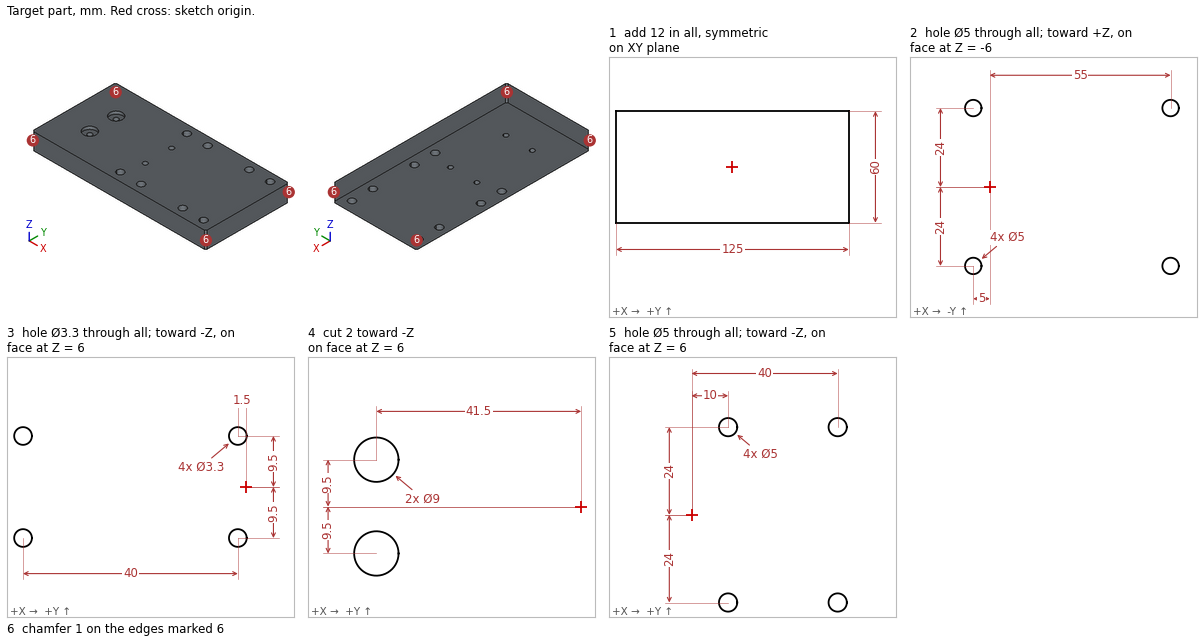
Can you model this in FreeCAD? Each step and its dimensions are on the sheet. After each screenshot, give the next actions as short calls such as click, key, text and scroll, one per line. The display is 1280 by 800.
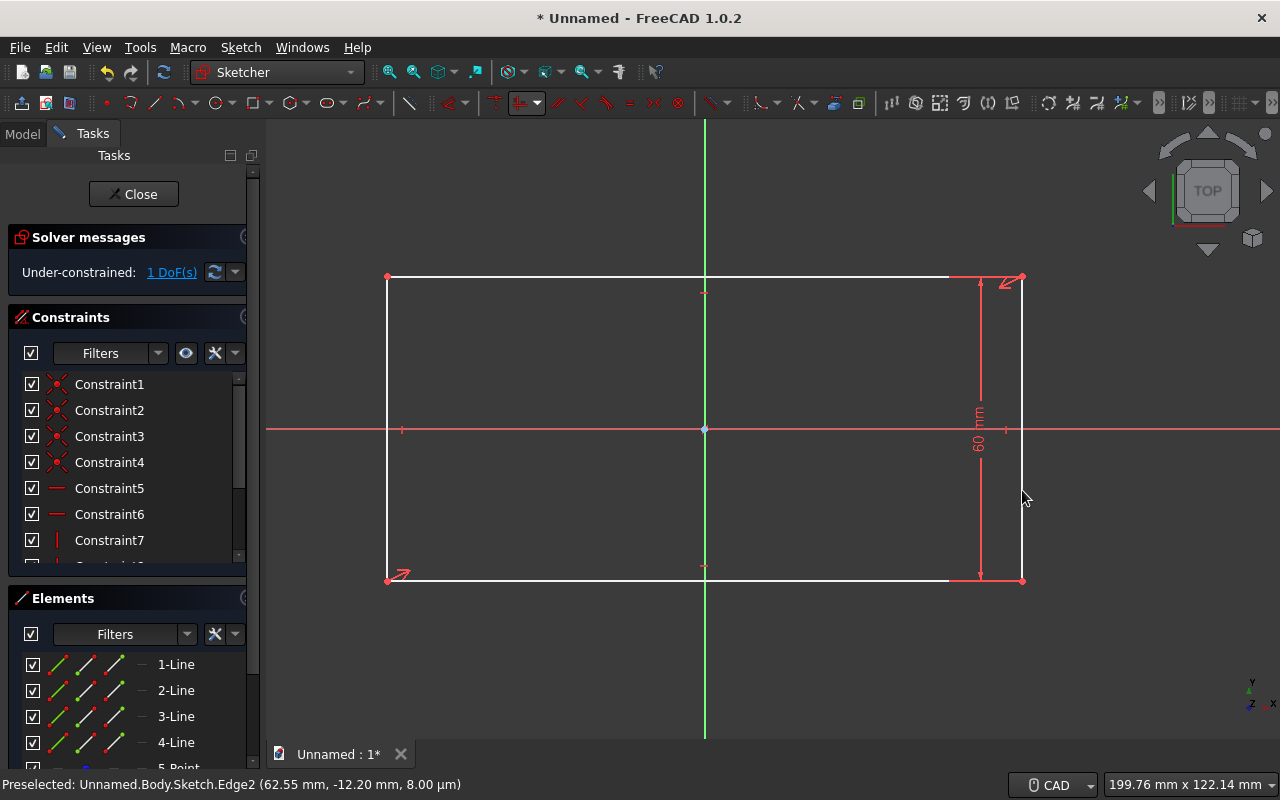
click(578, 581)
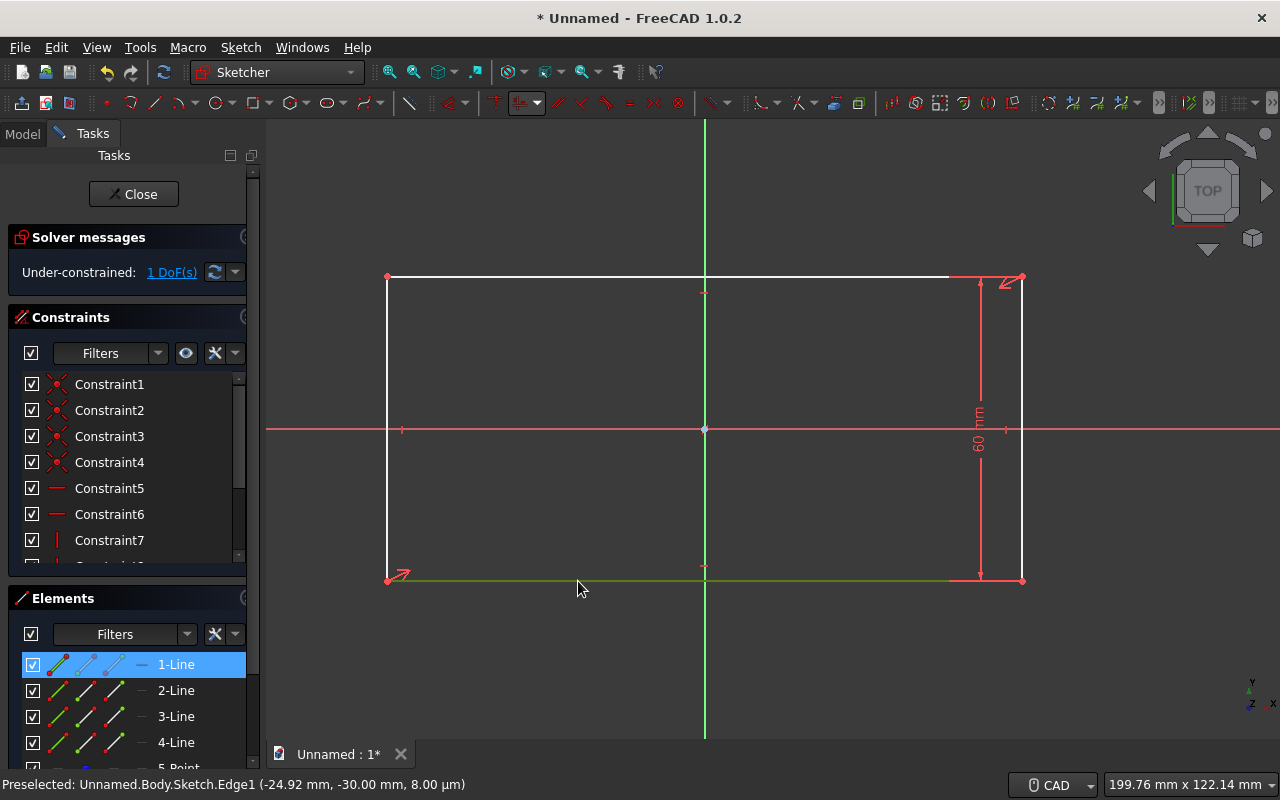
key(l)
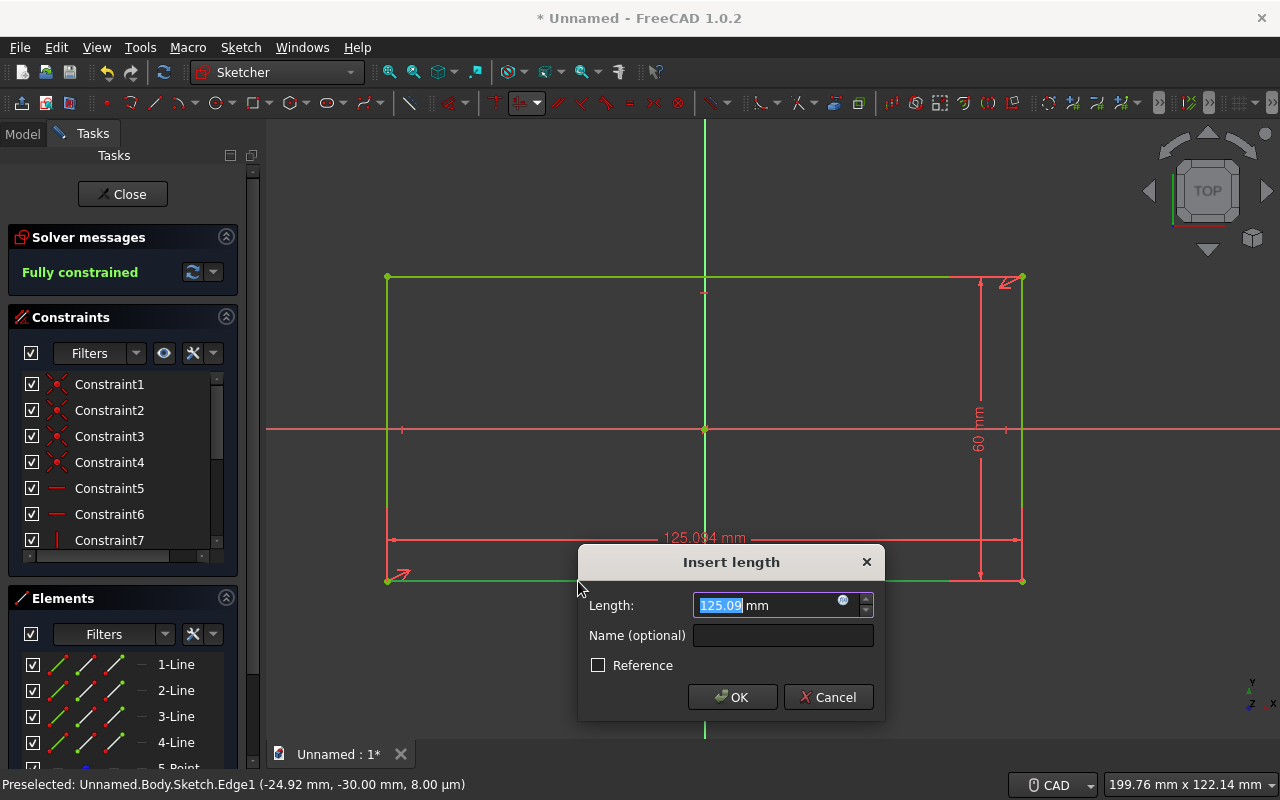
text(125)
key(Return)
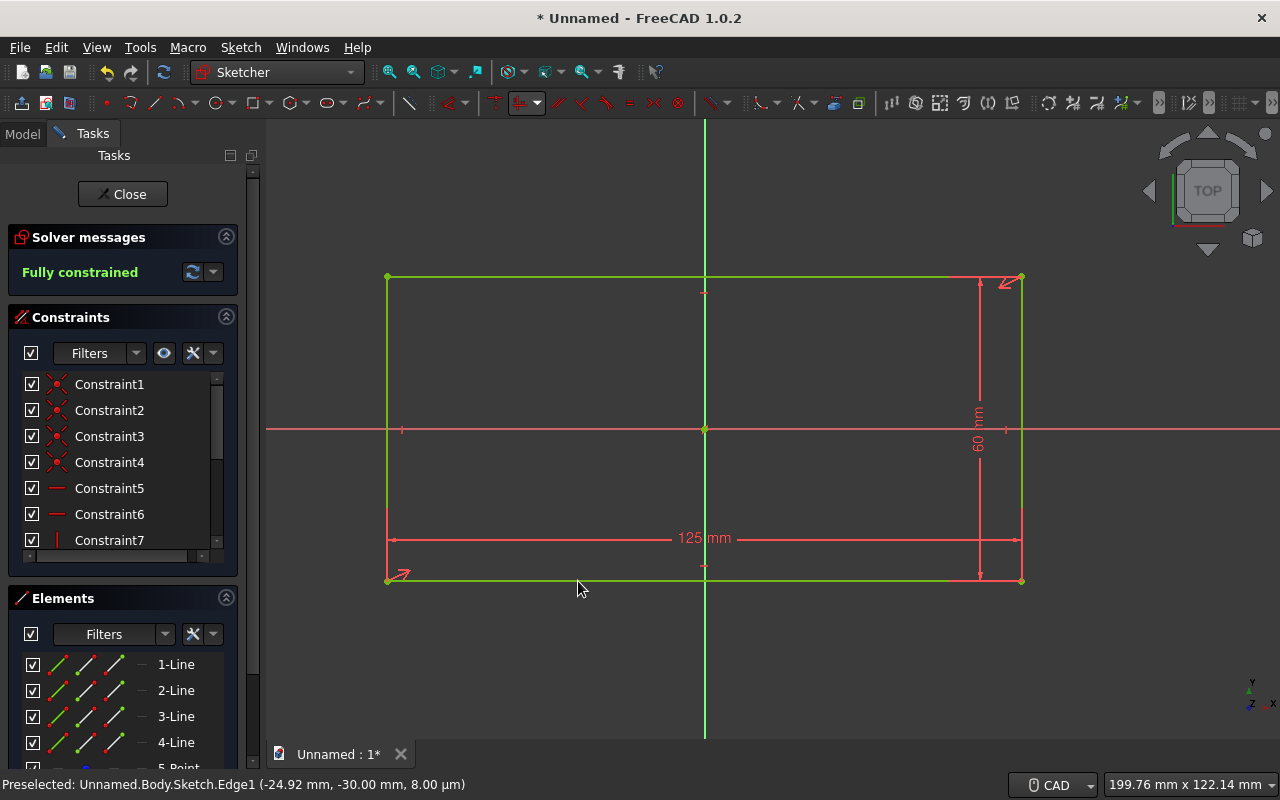
click(123, 194)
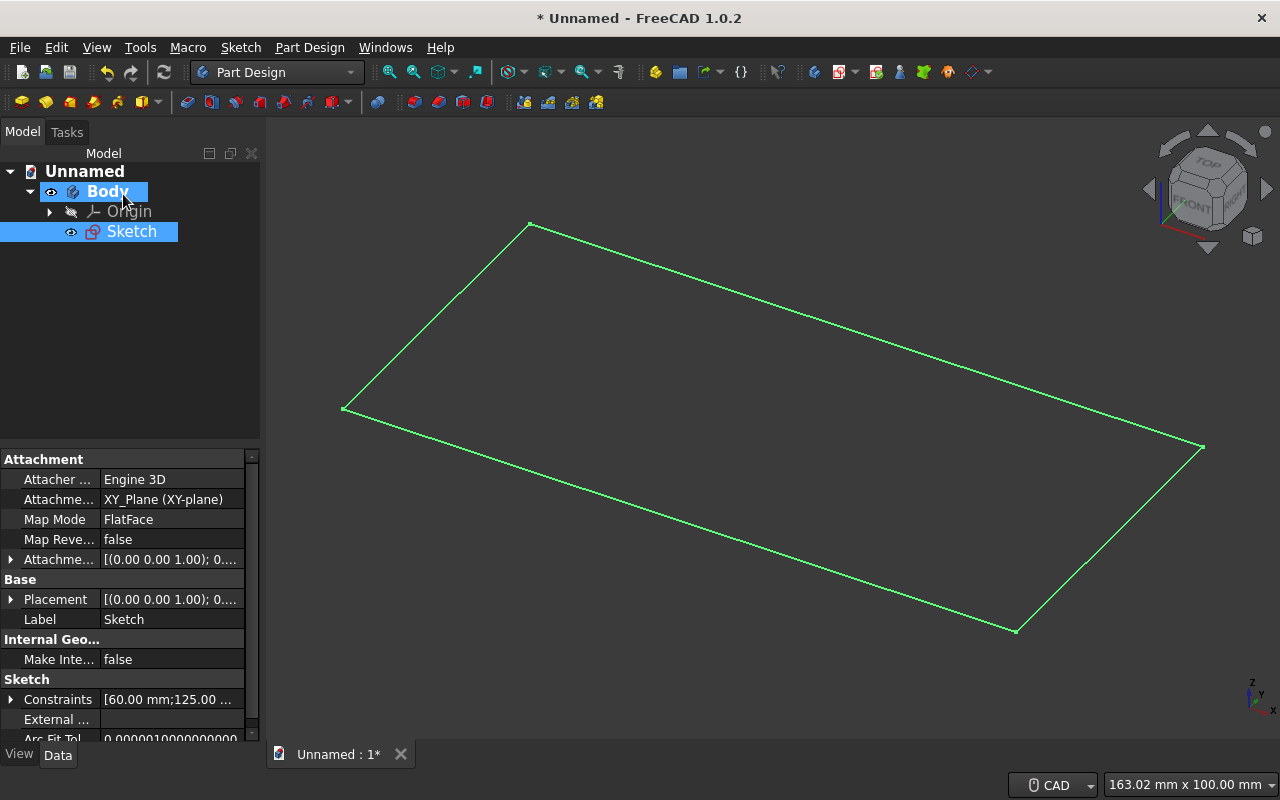
click(22, 102)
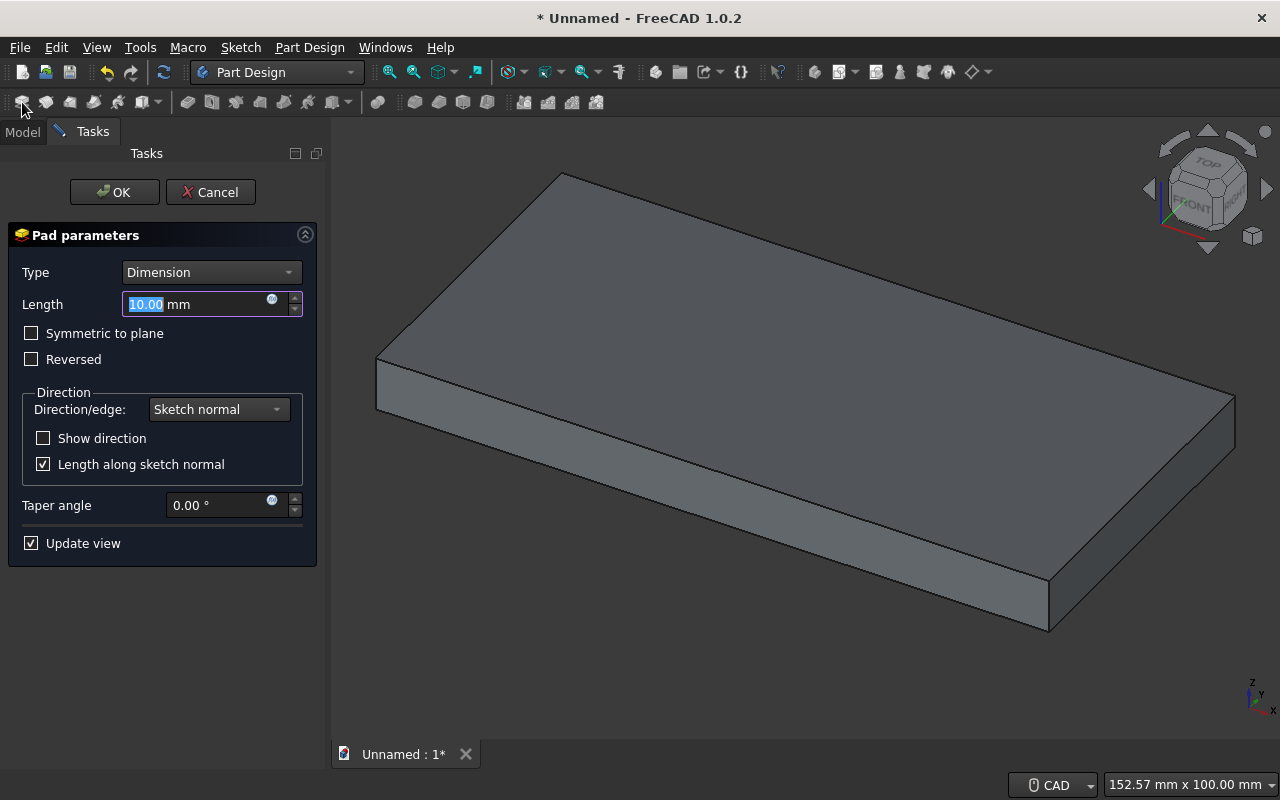
text(12)
key(Tab)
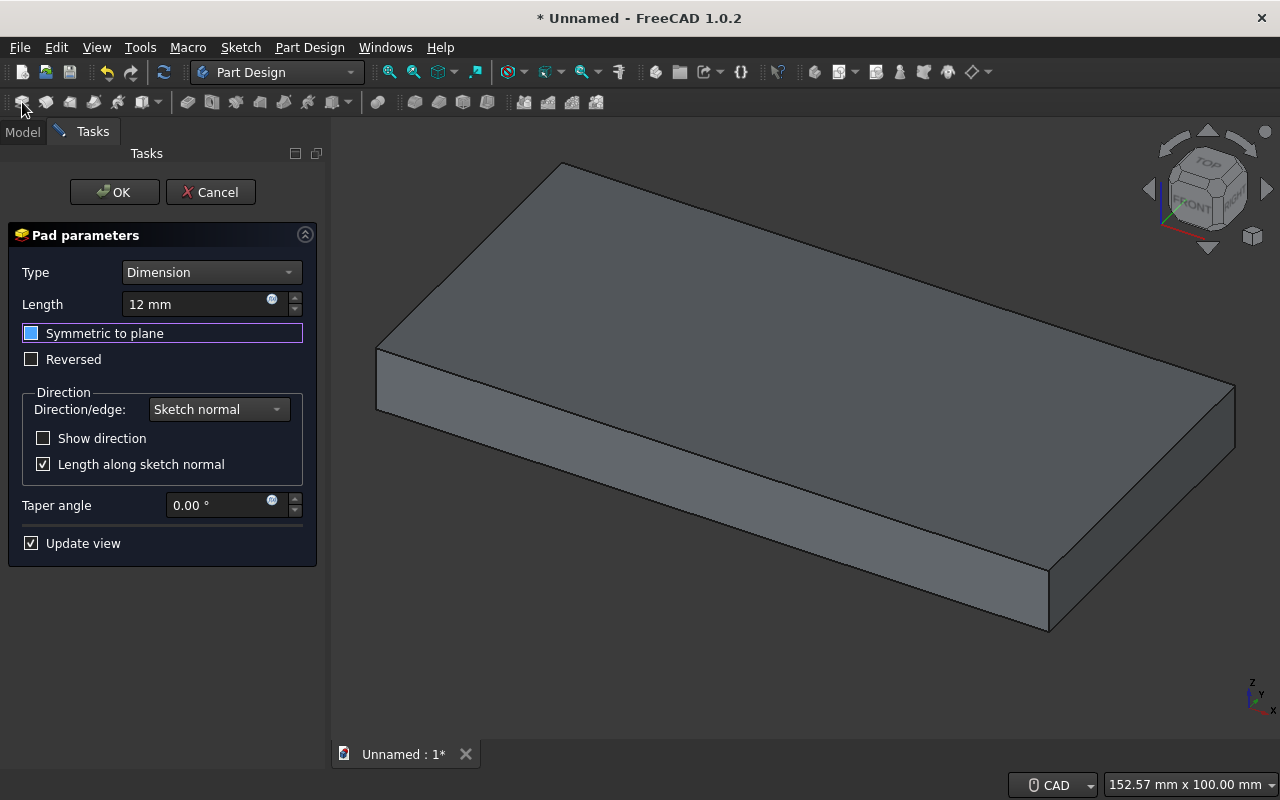
click(30, 333)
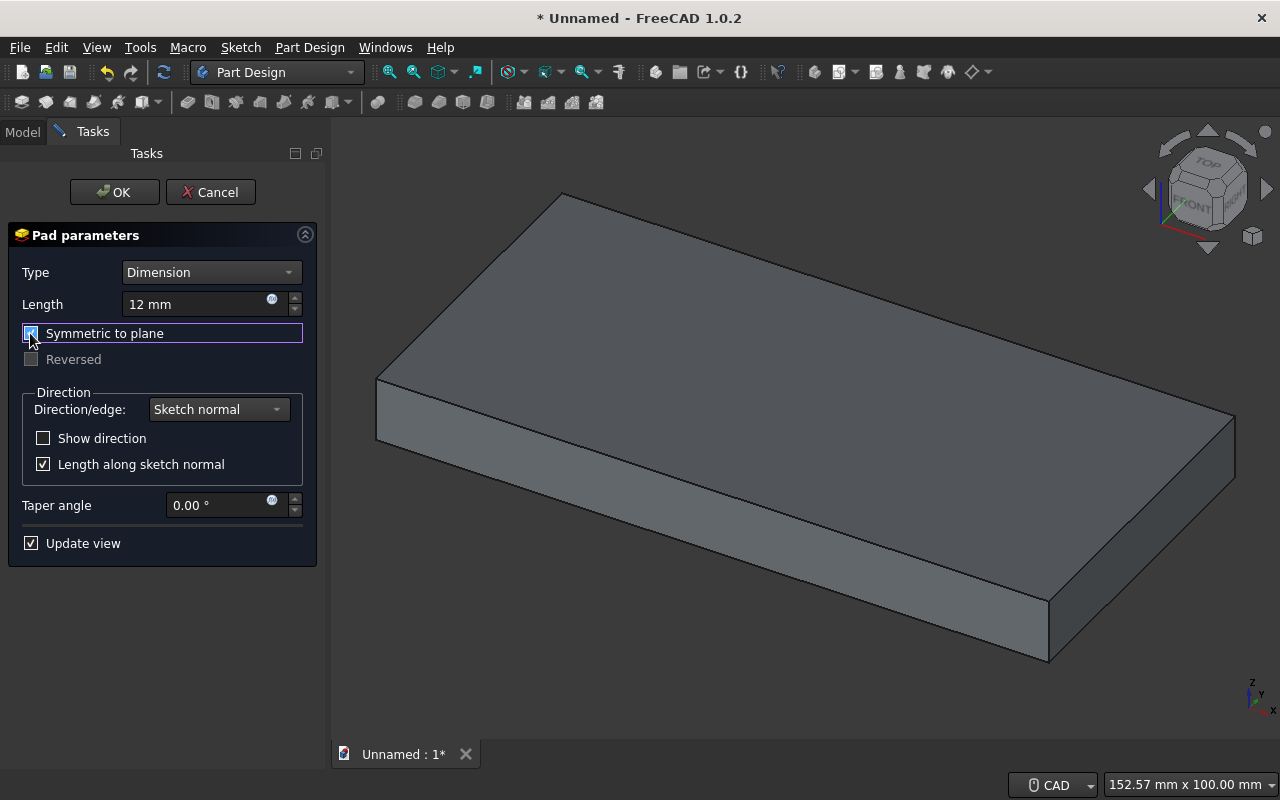
click(115, 192)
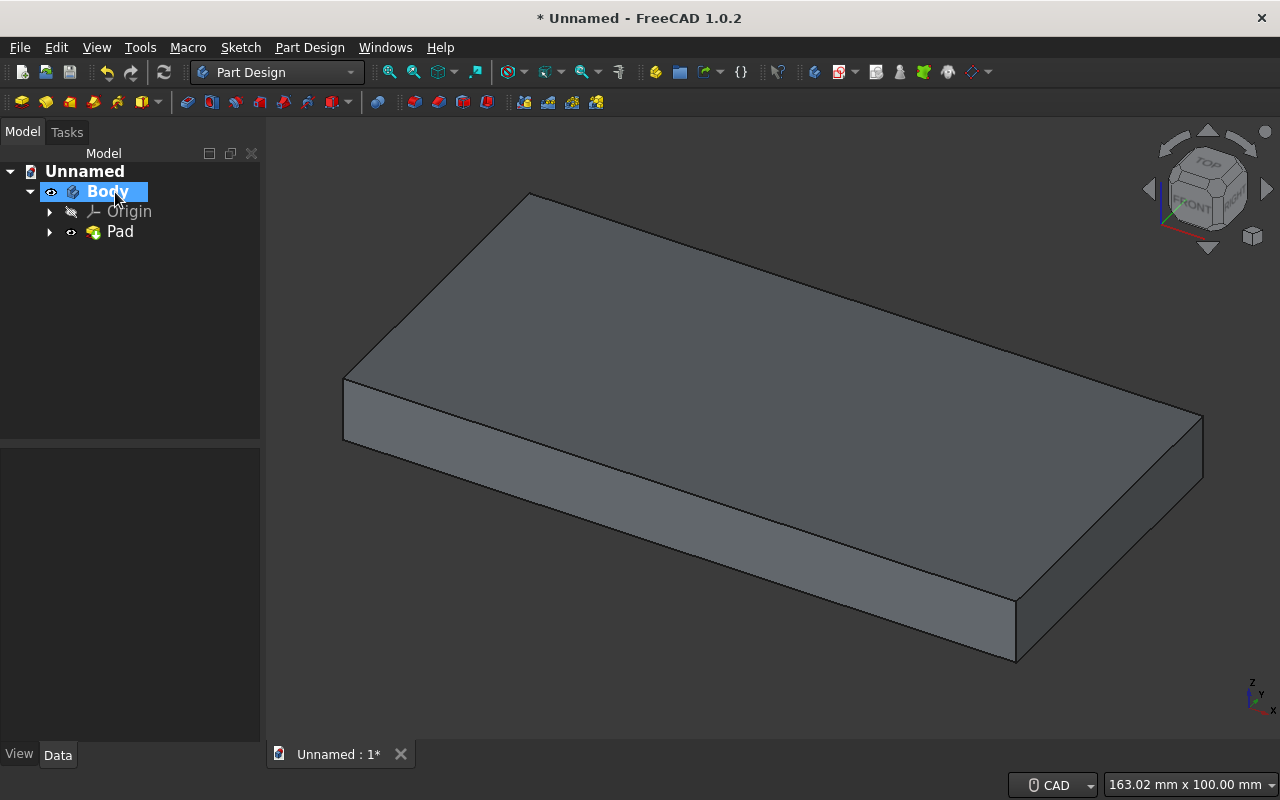
key(5)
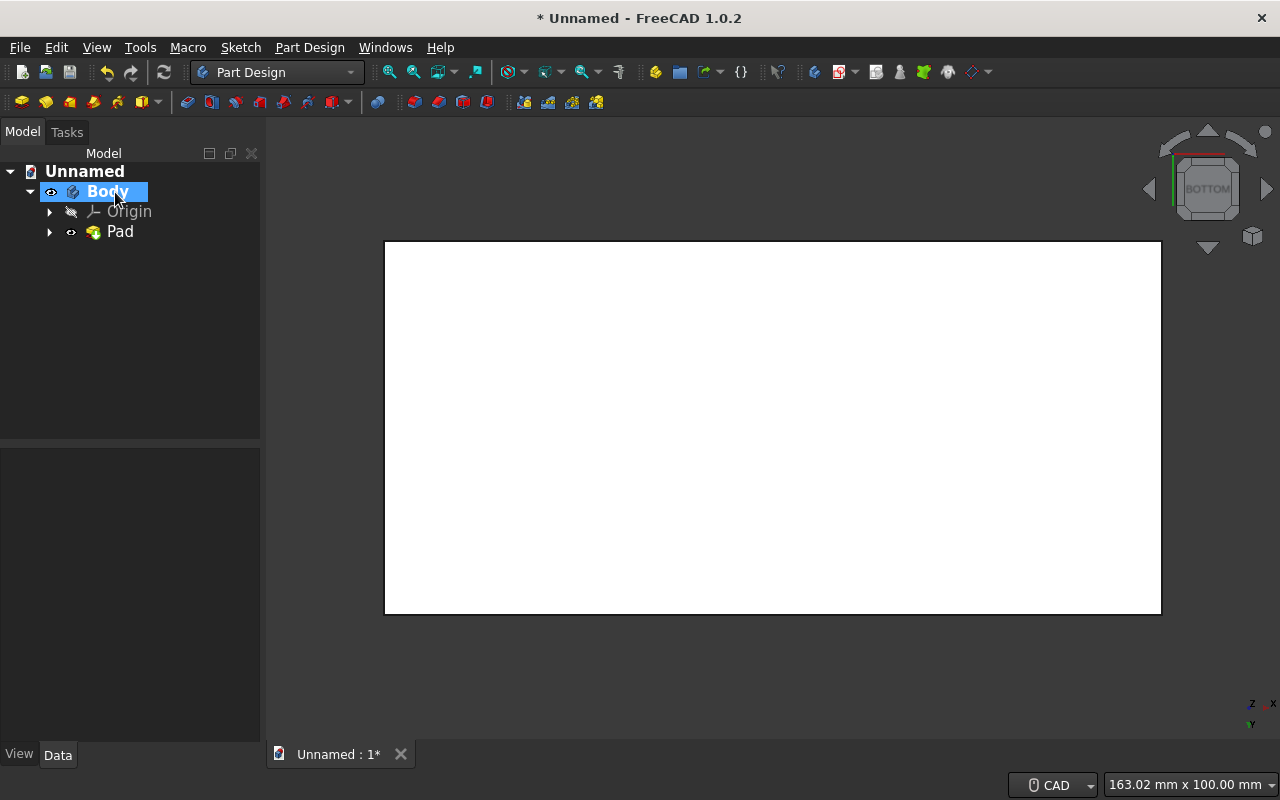
click(884, 427)